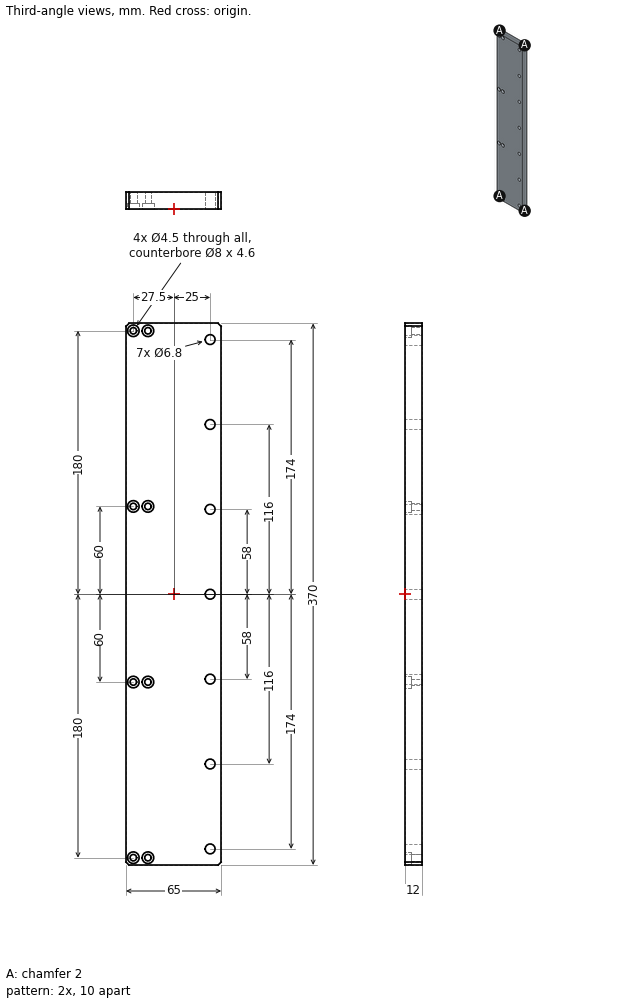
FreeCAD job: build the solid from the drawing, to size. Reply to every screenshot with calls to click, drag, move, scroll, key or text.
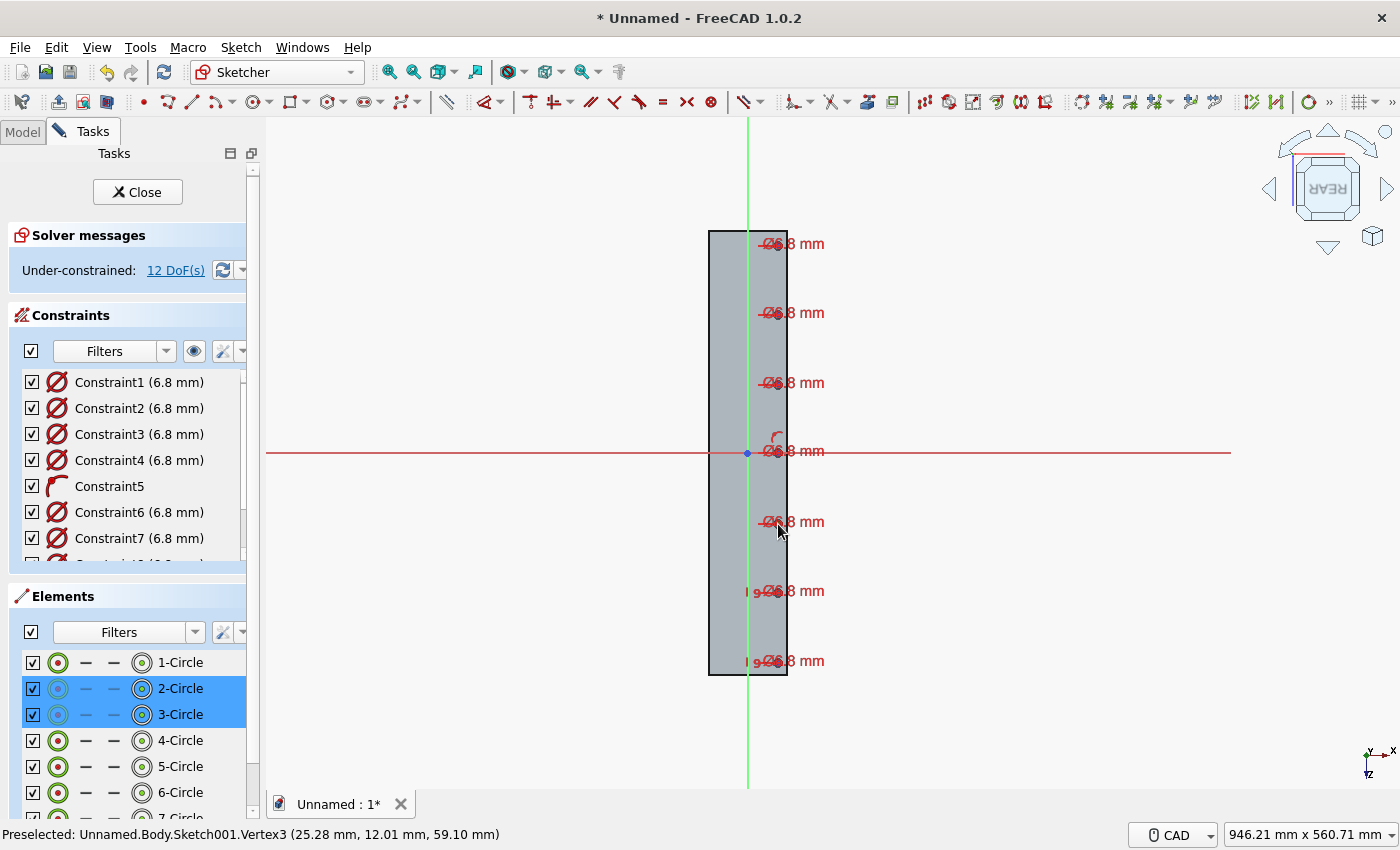
key(v)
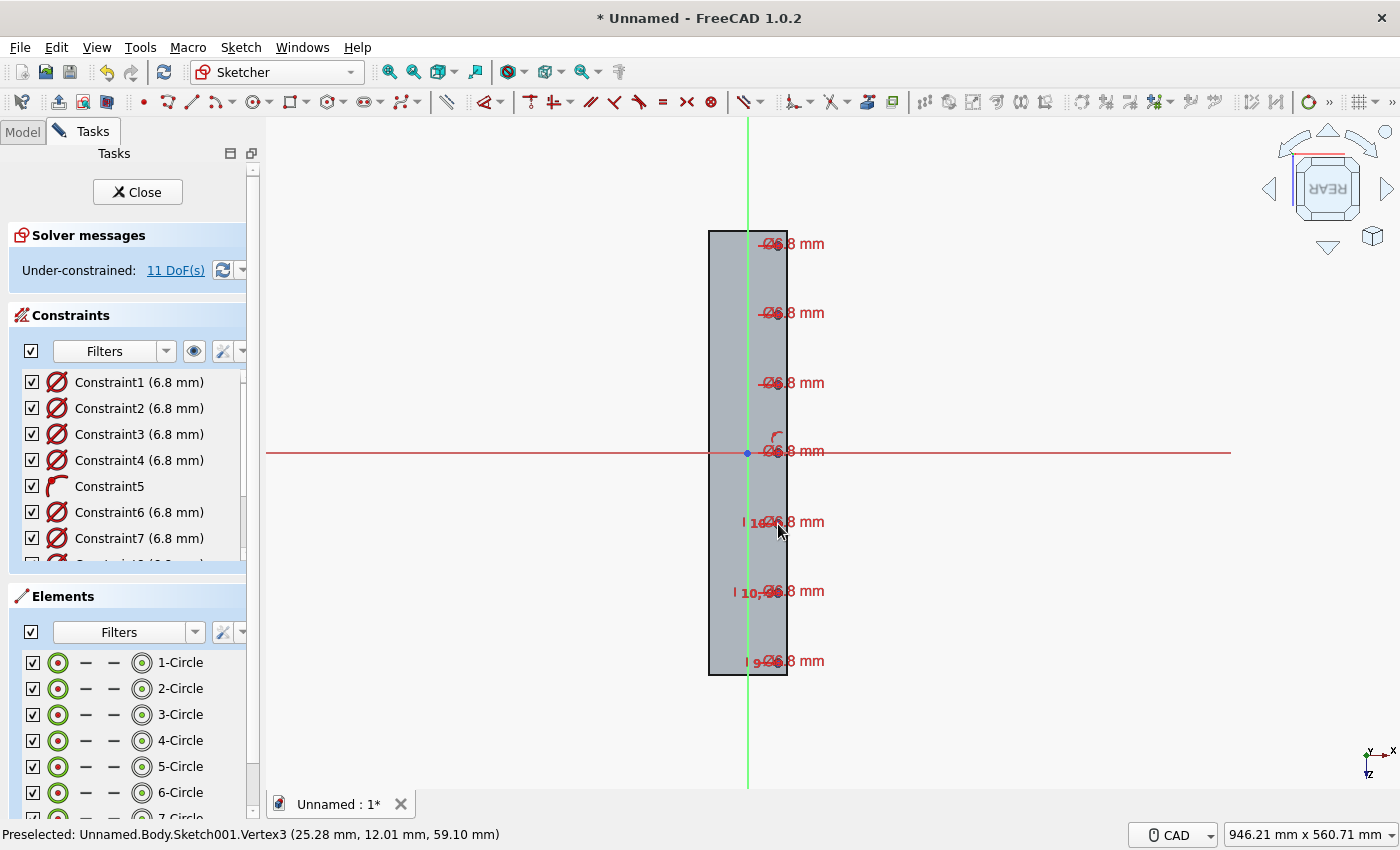
click(778, 524)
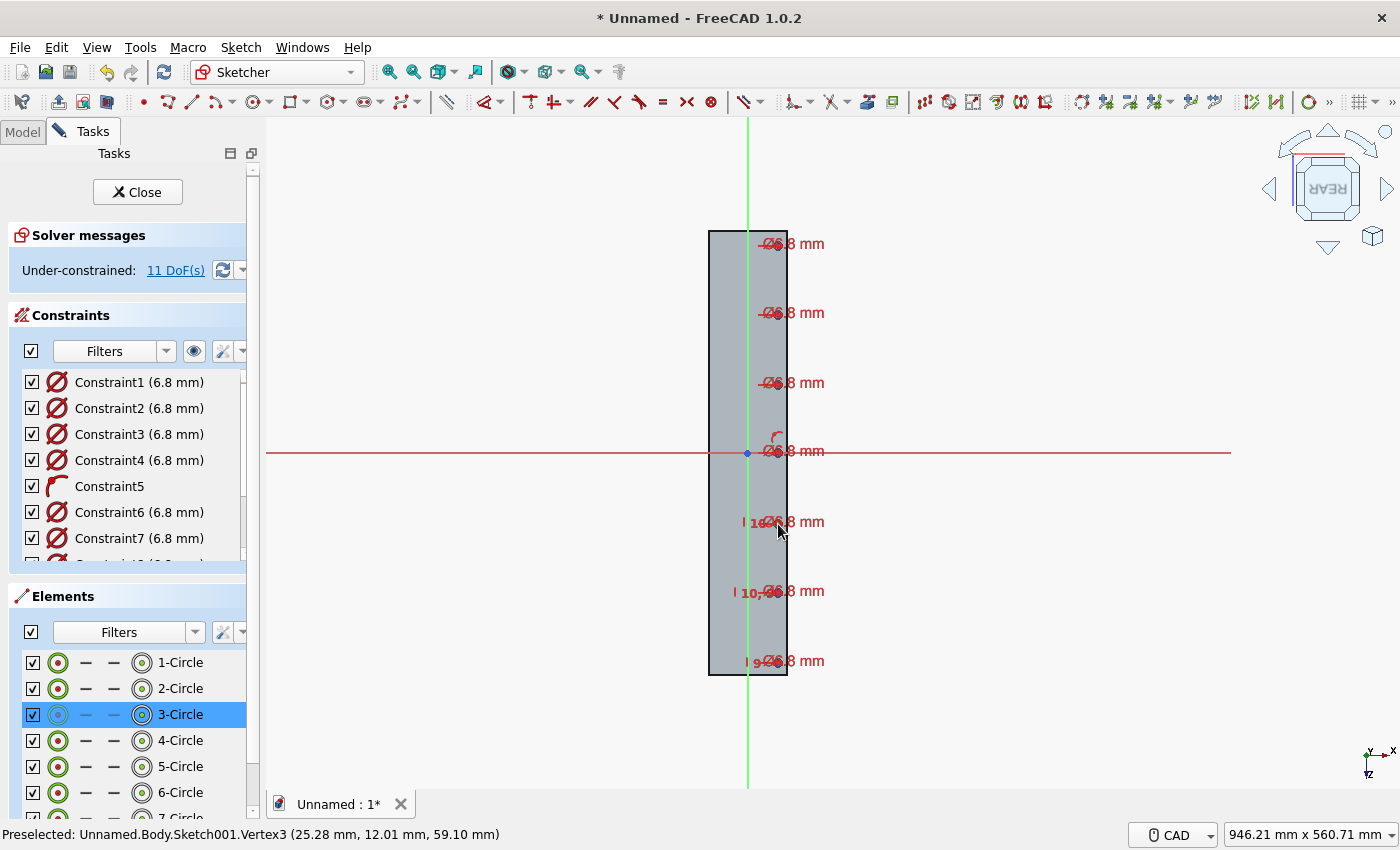
click(778, 453)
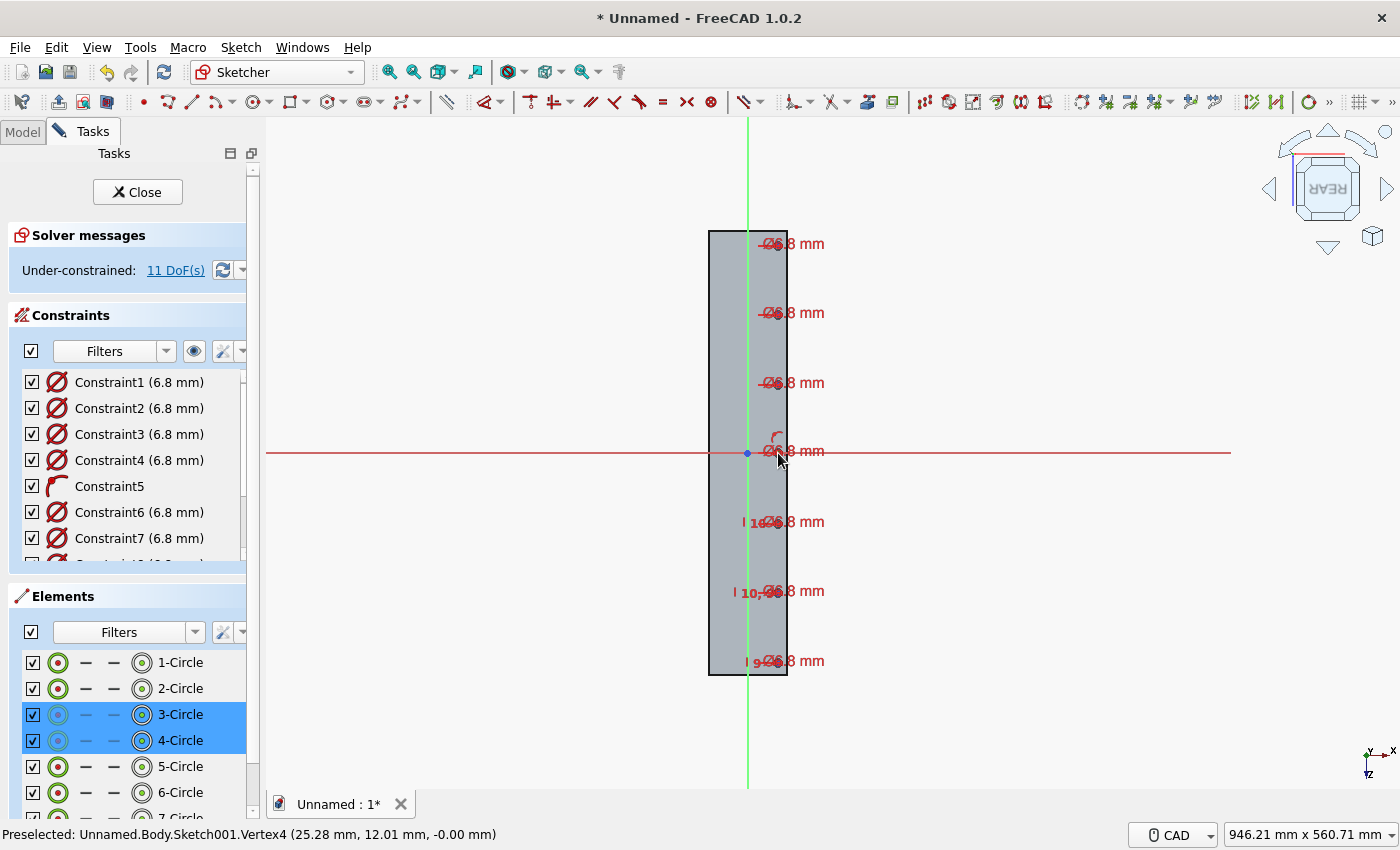
key(v)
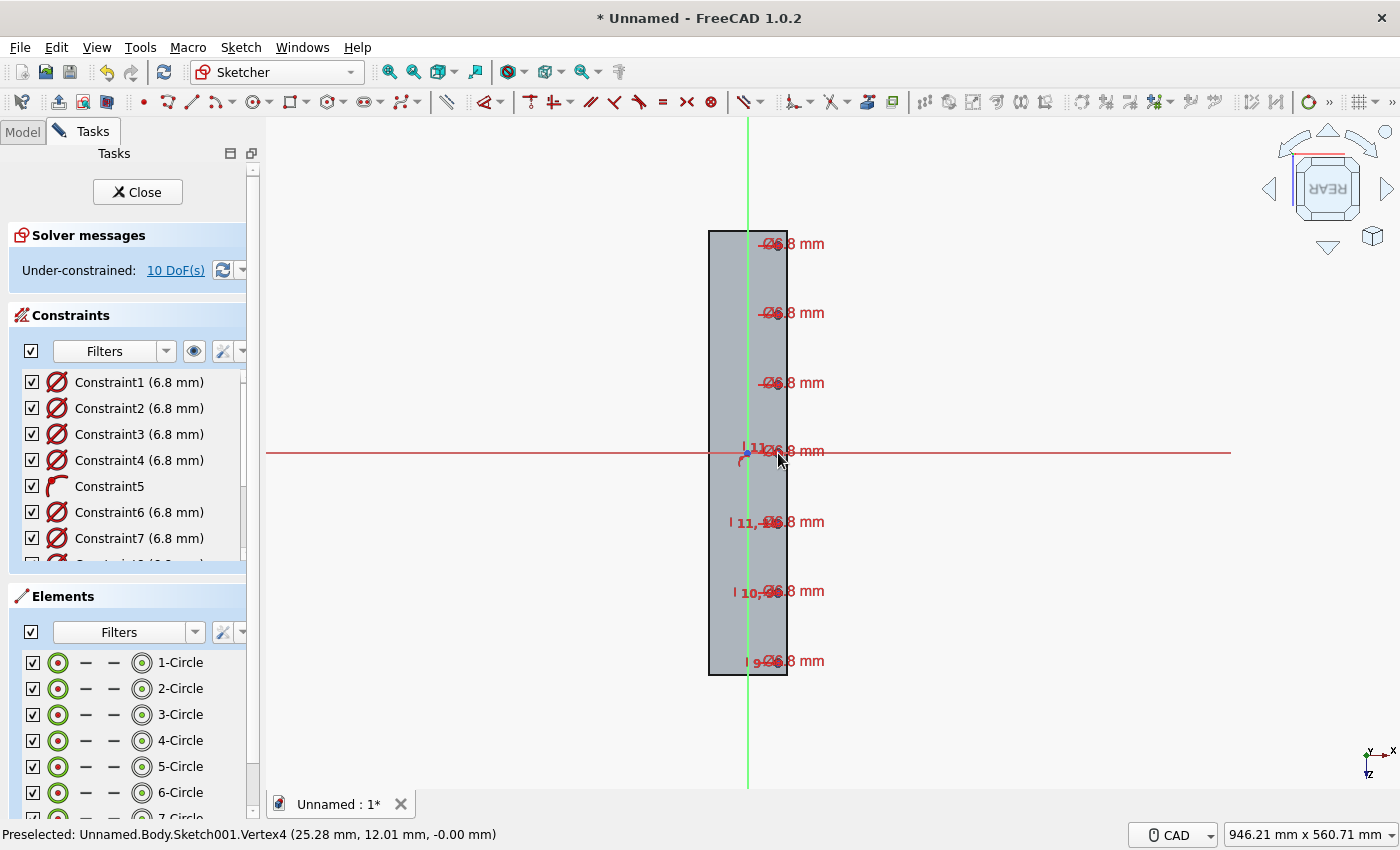
click(778, 453)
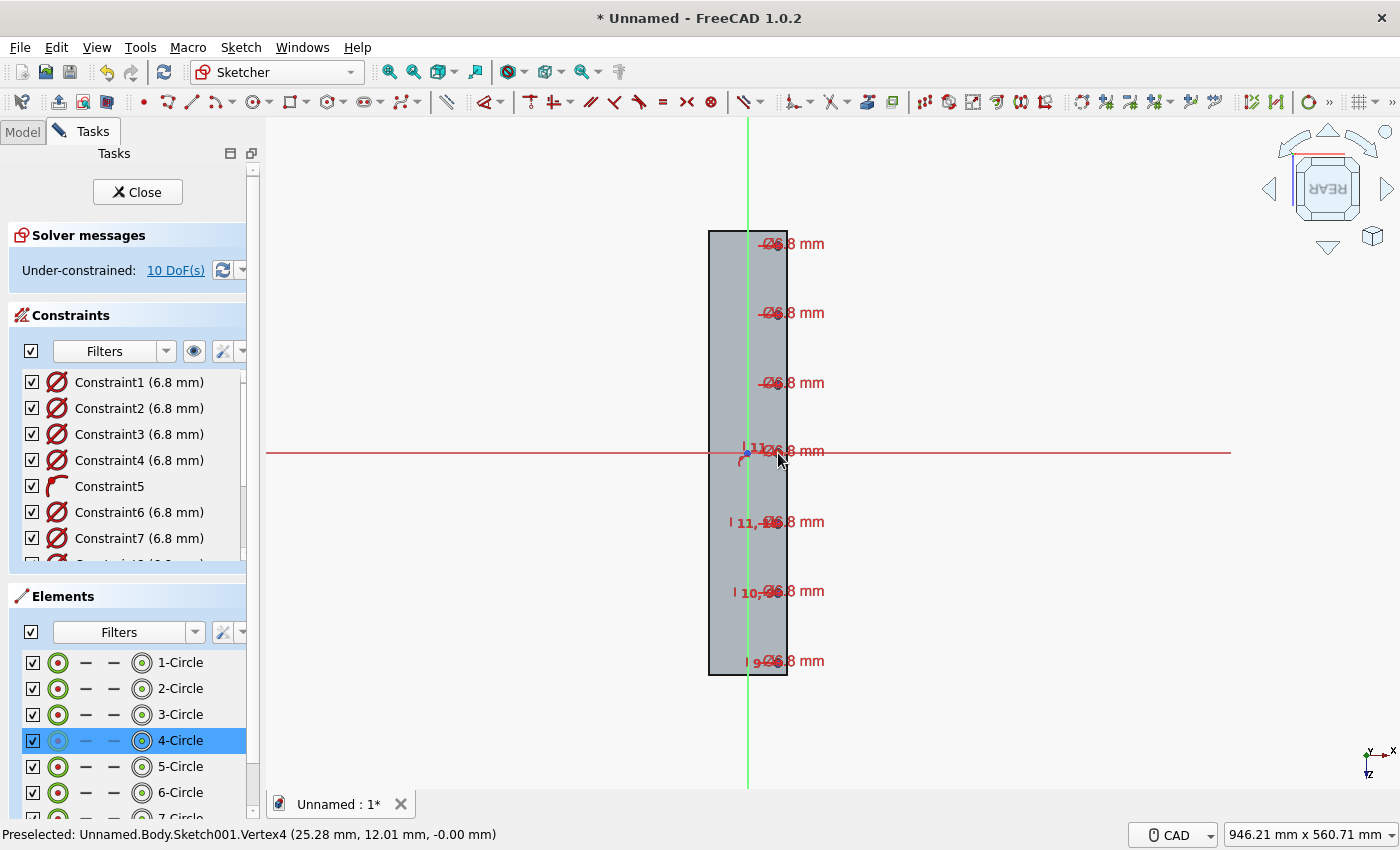
click(778, 385)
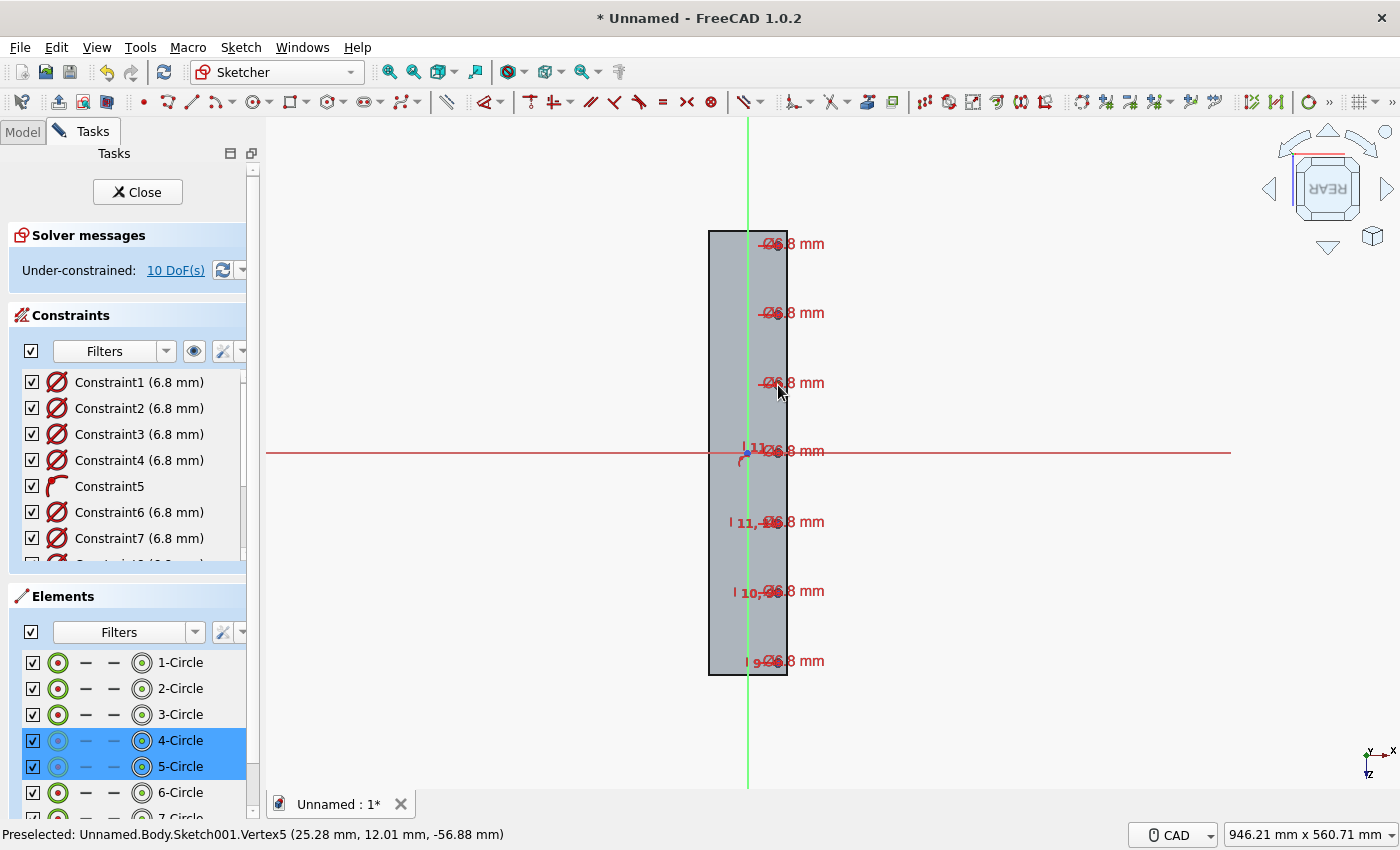
click(572, 102)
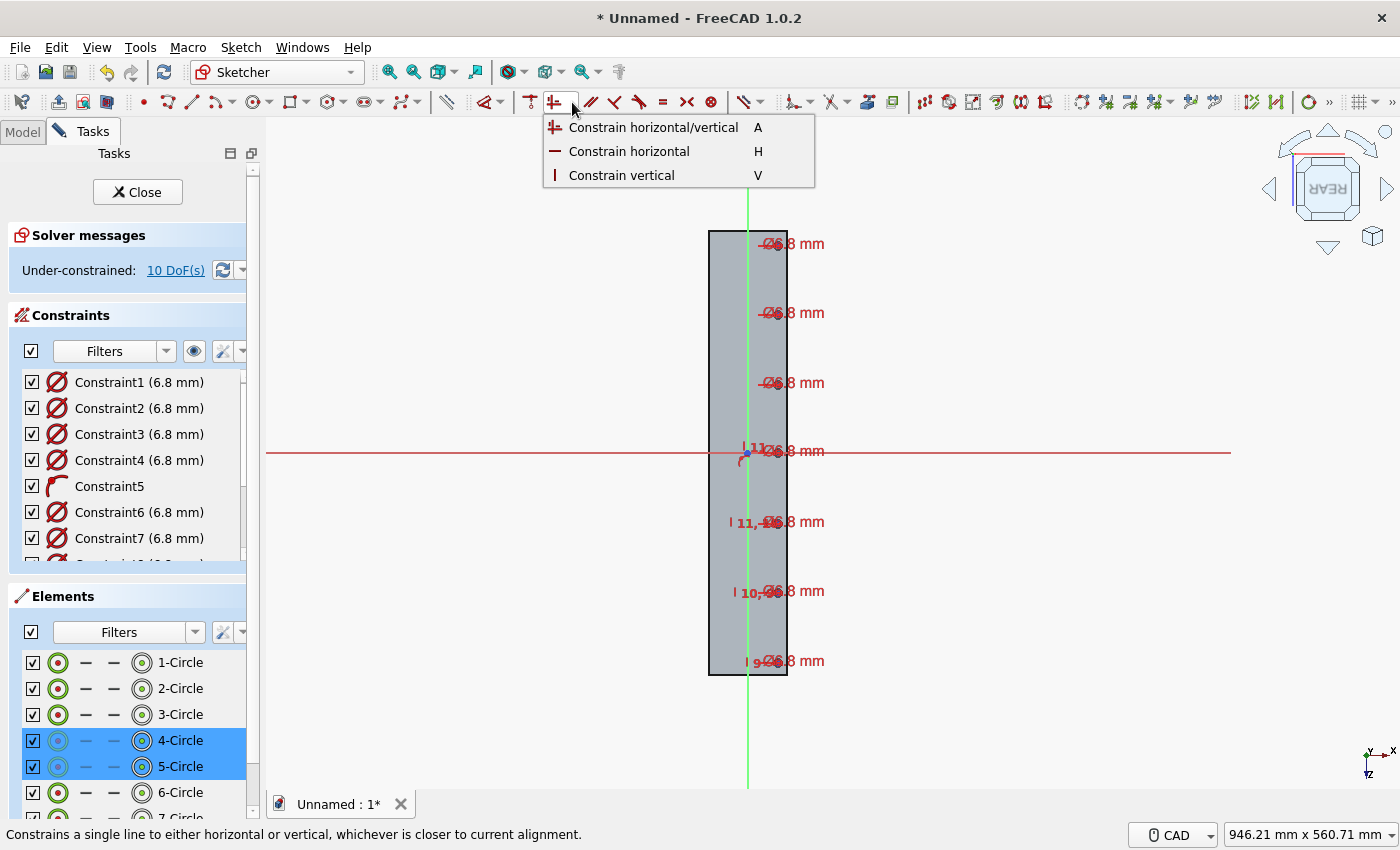
click(679, 175)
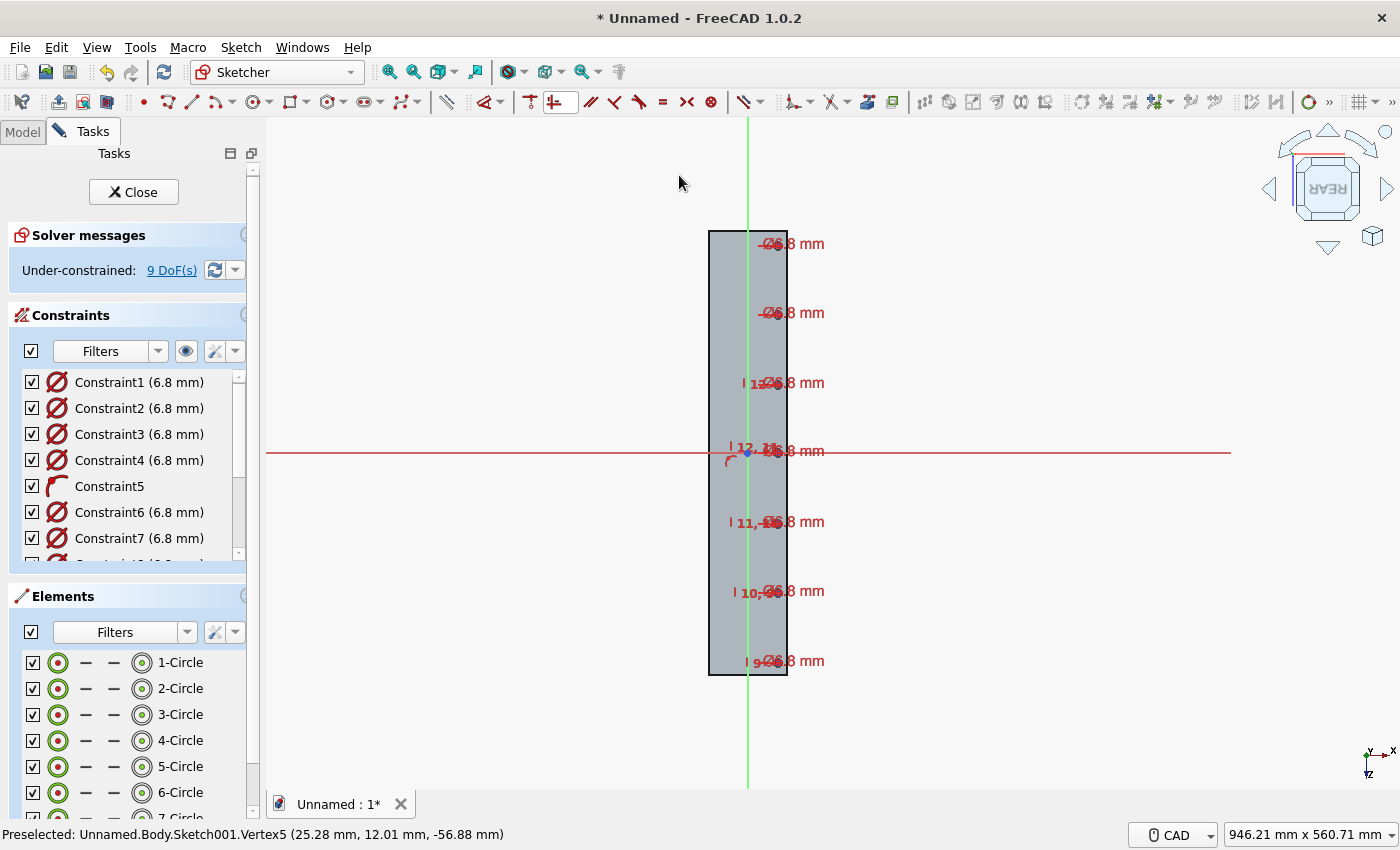
click(778, 385)